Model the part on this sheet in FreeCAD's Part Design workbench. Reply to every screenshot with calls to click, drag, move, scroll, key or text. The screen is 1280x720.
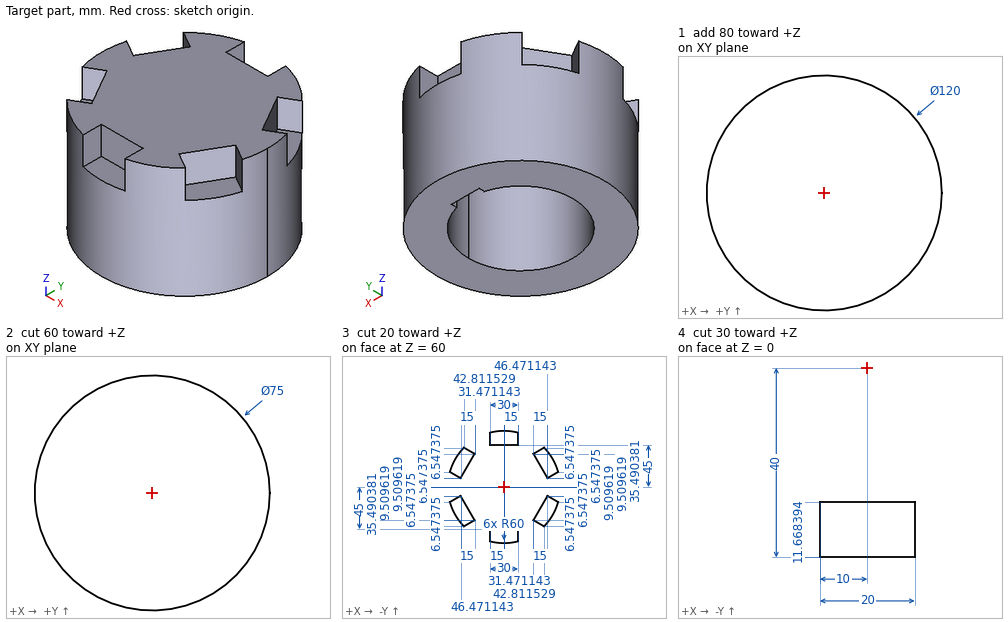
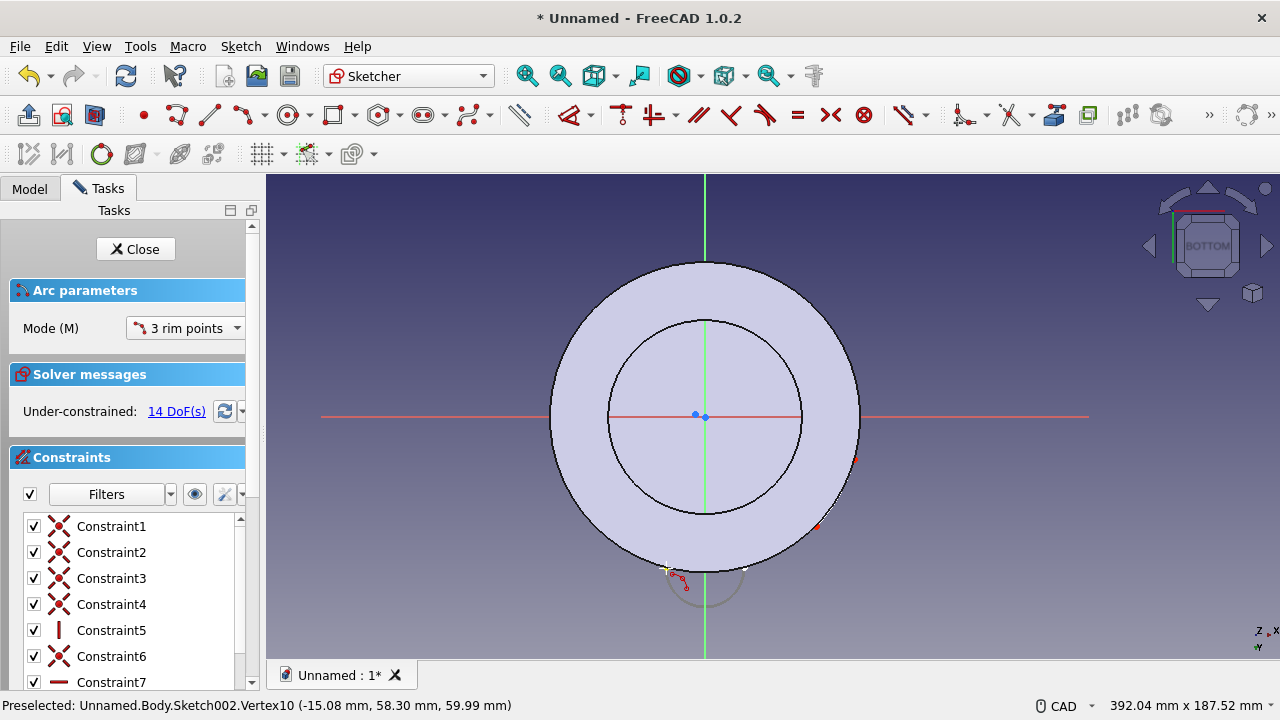
scroll(697, 572, up, 7)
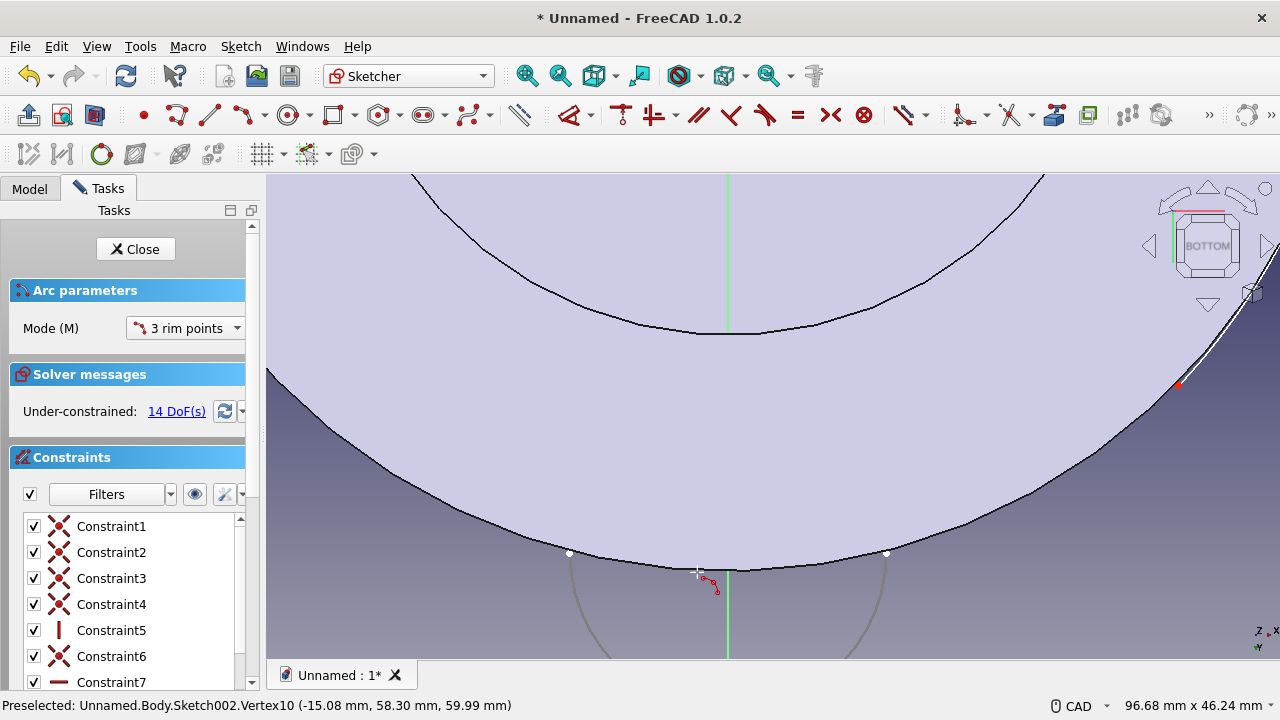
click(696, 570)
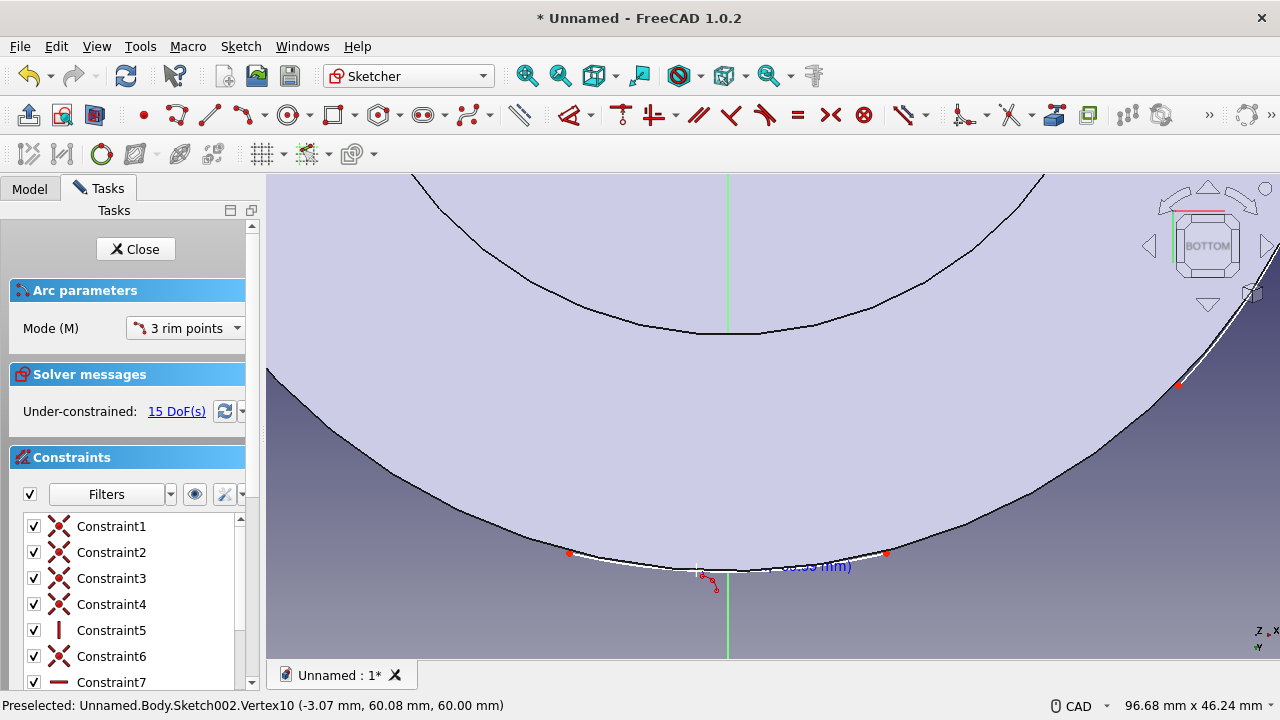
click(177, 116)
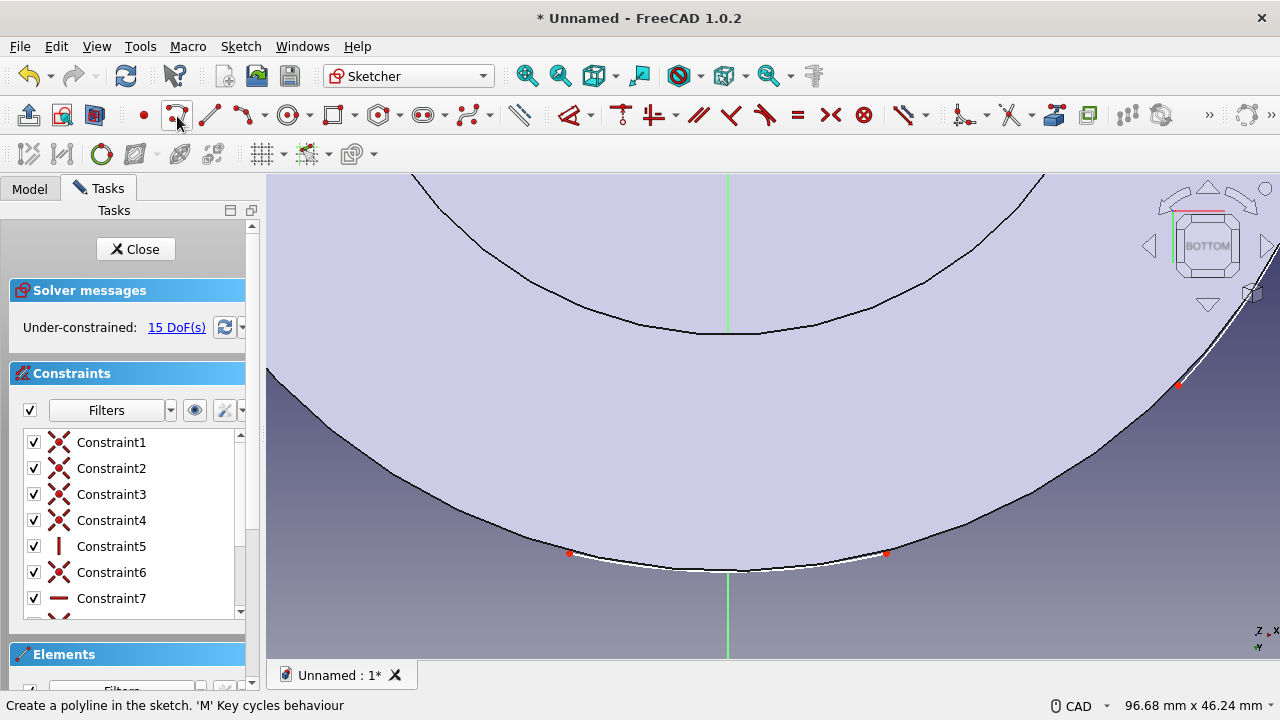
scroll(697, 572, down, 7)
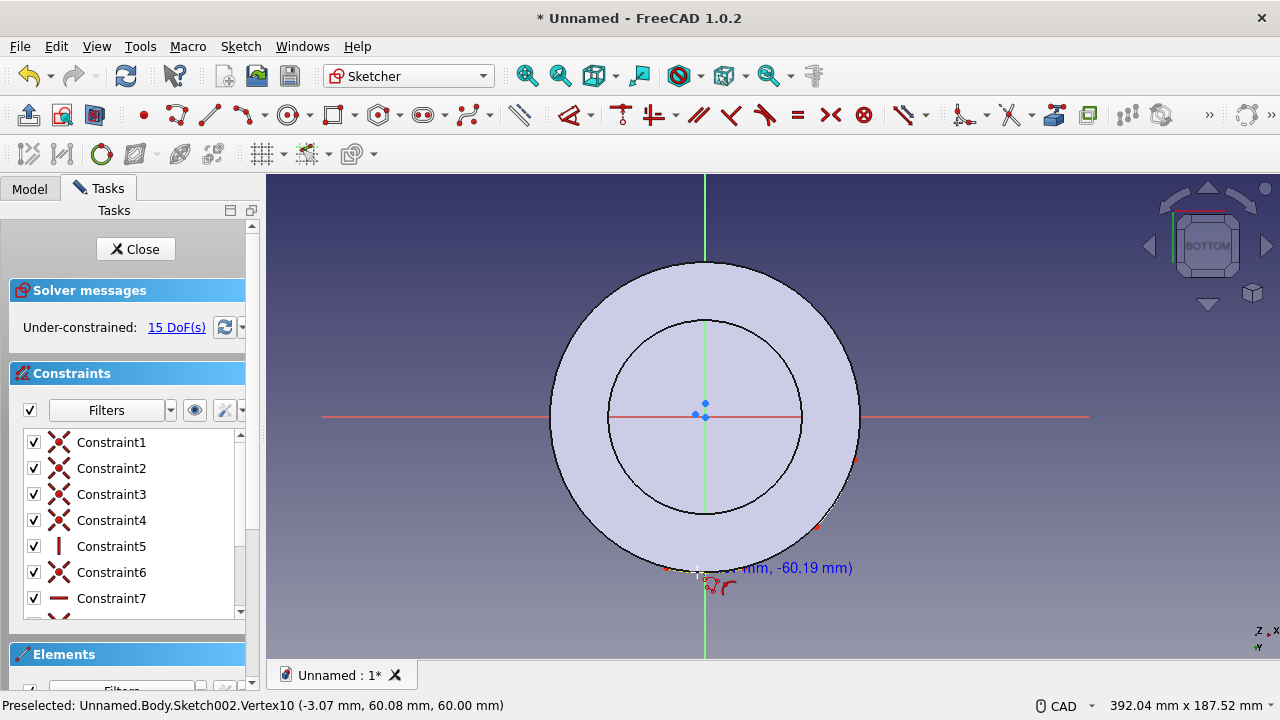
click(855, 376)
click(825, 393)
click(786, 325)
click(816, 308)
right_click(816, 308)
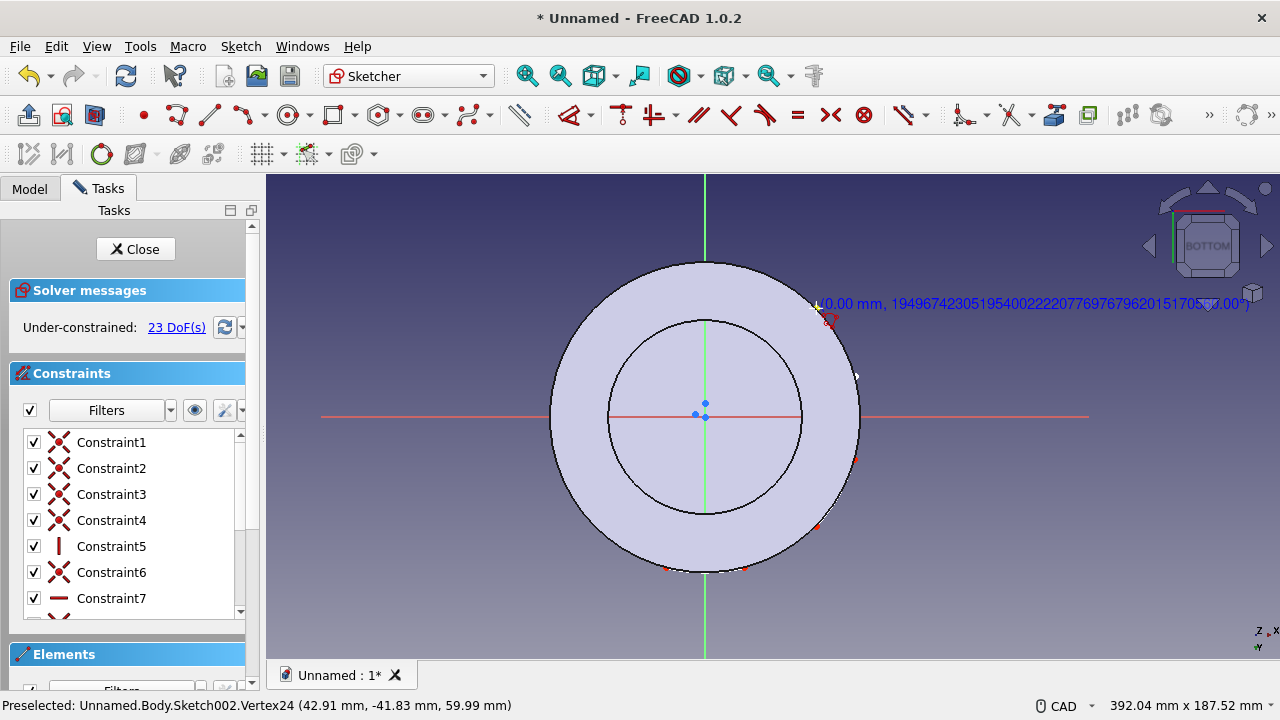
click(242, 116)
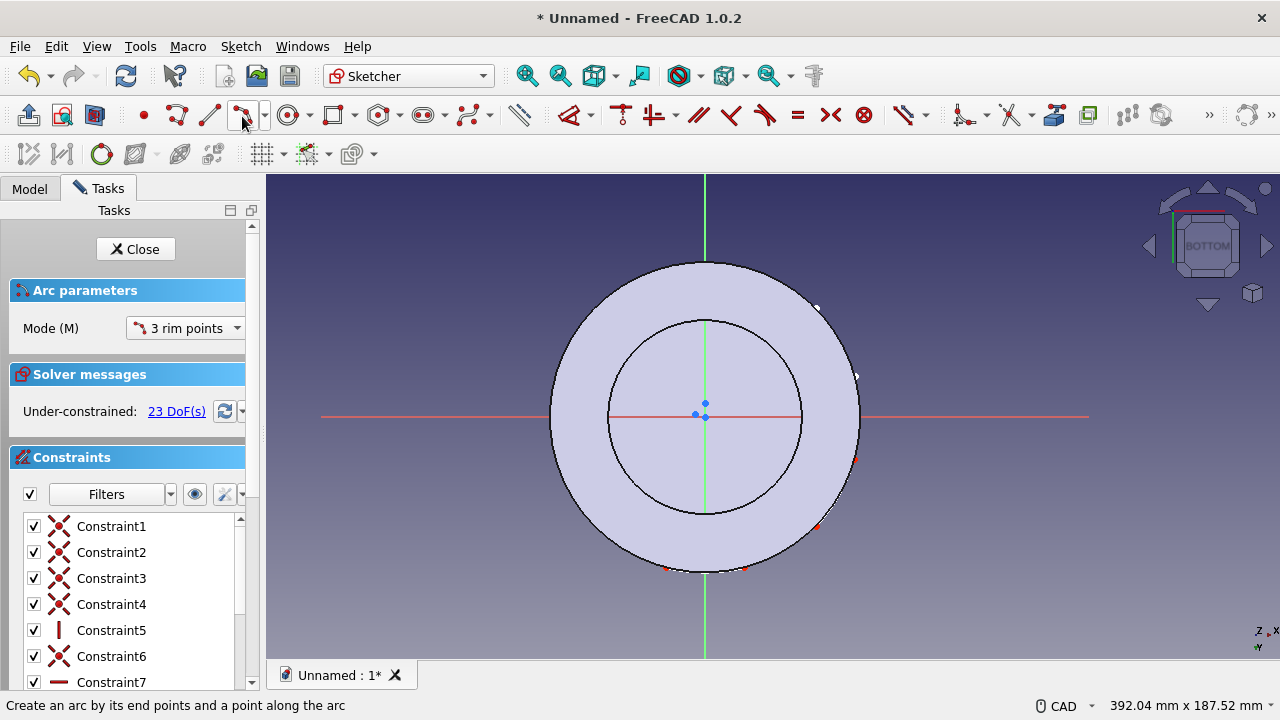
click(816, 309)
click(855, 377)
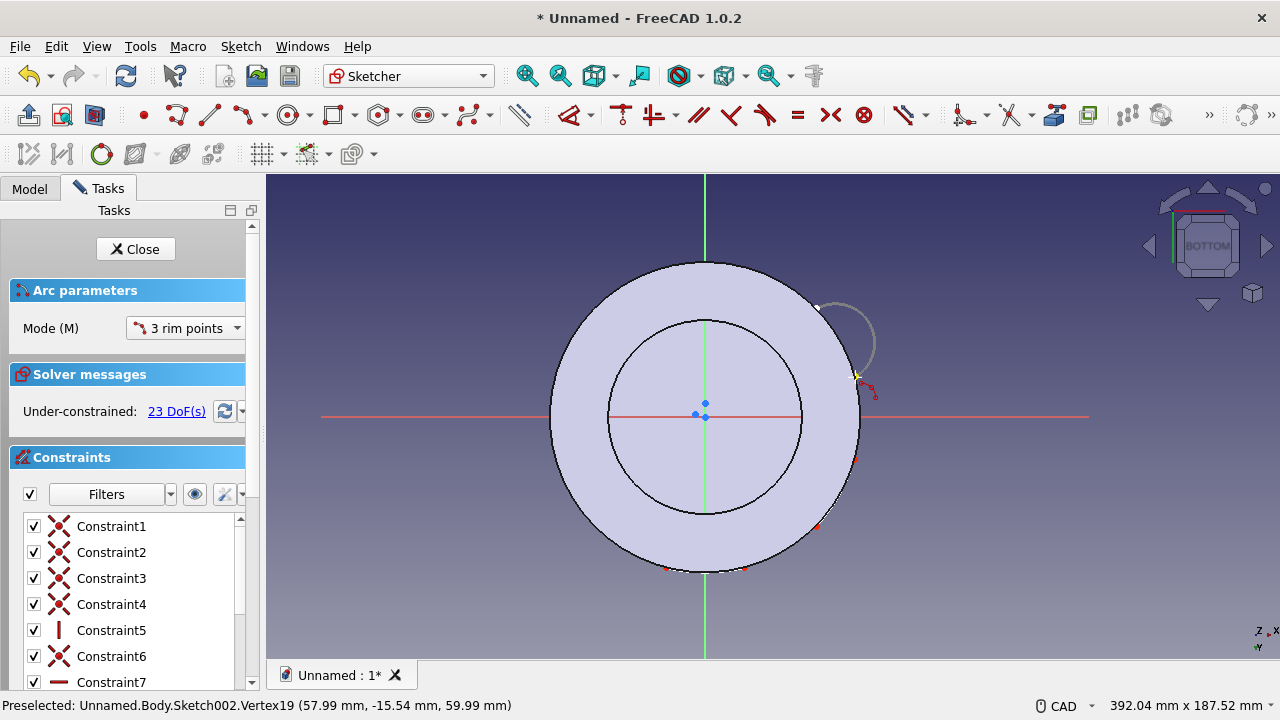
scroll(839, 340, up, 6)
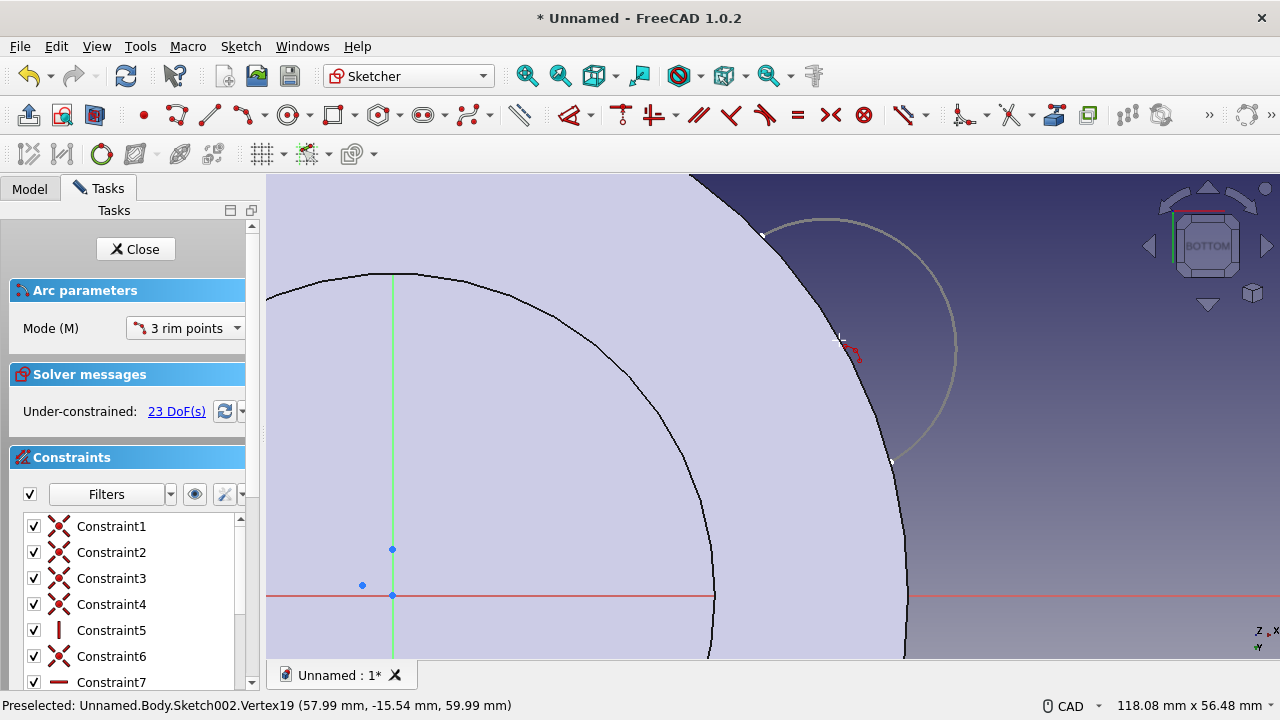
click(839, 338)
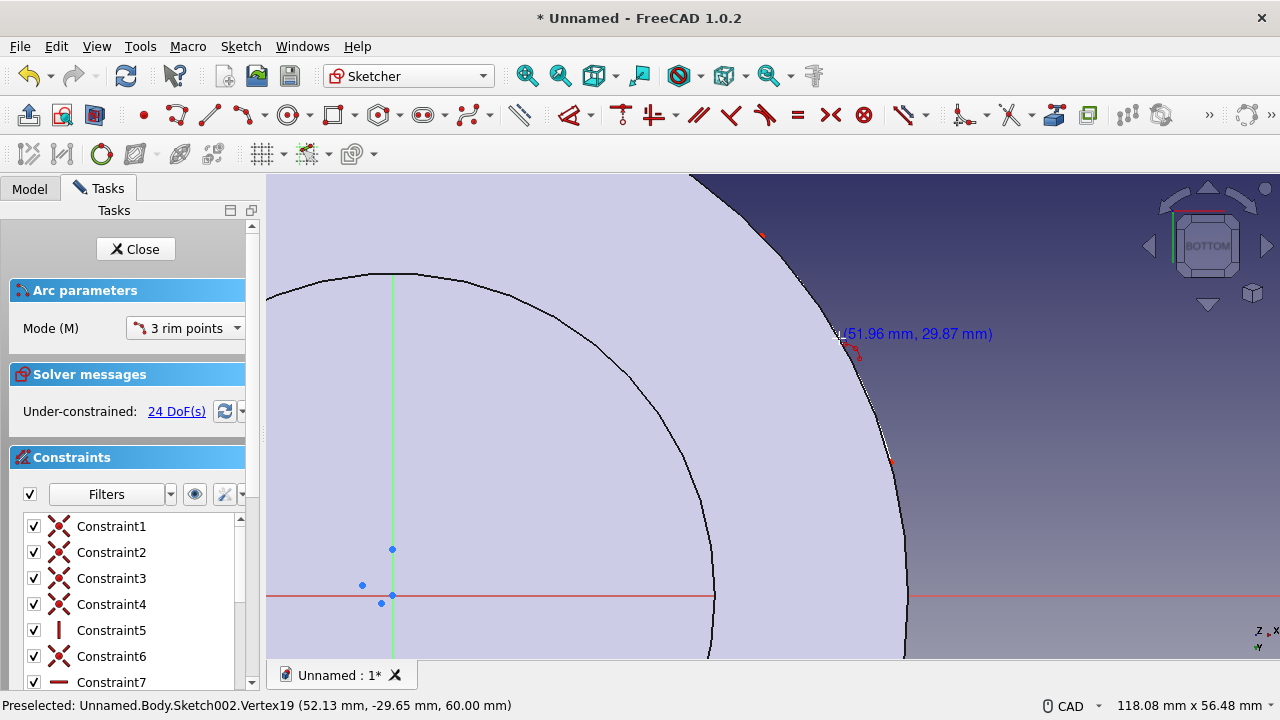
click(177, 116)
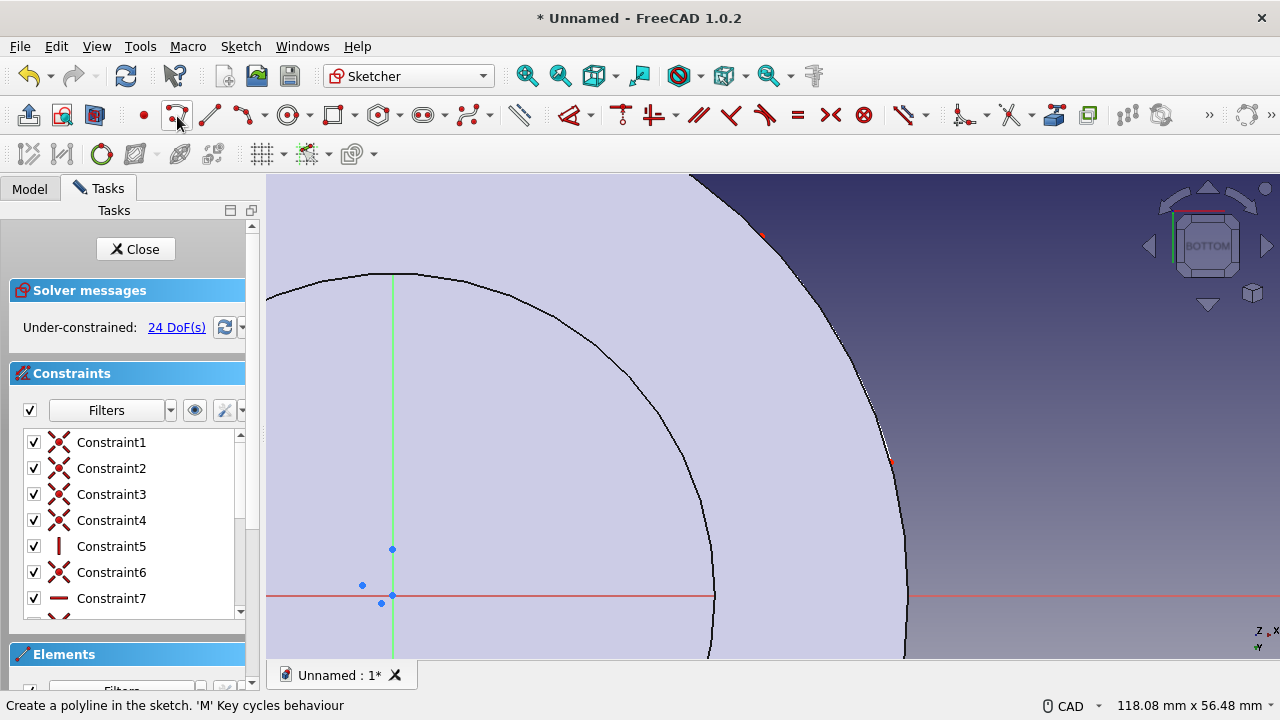
scroll(839, 339, down, 6)